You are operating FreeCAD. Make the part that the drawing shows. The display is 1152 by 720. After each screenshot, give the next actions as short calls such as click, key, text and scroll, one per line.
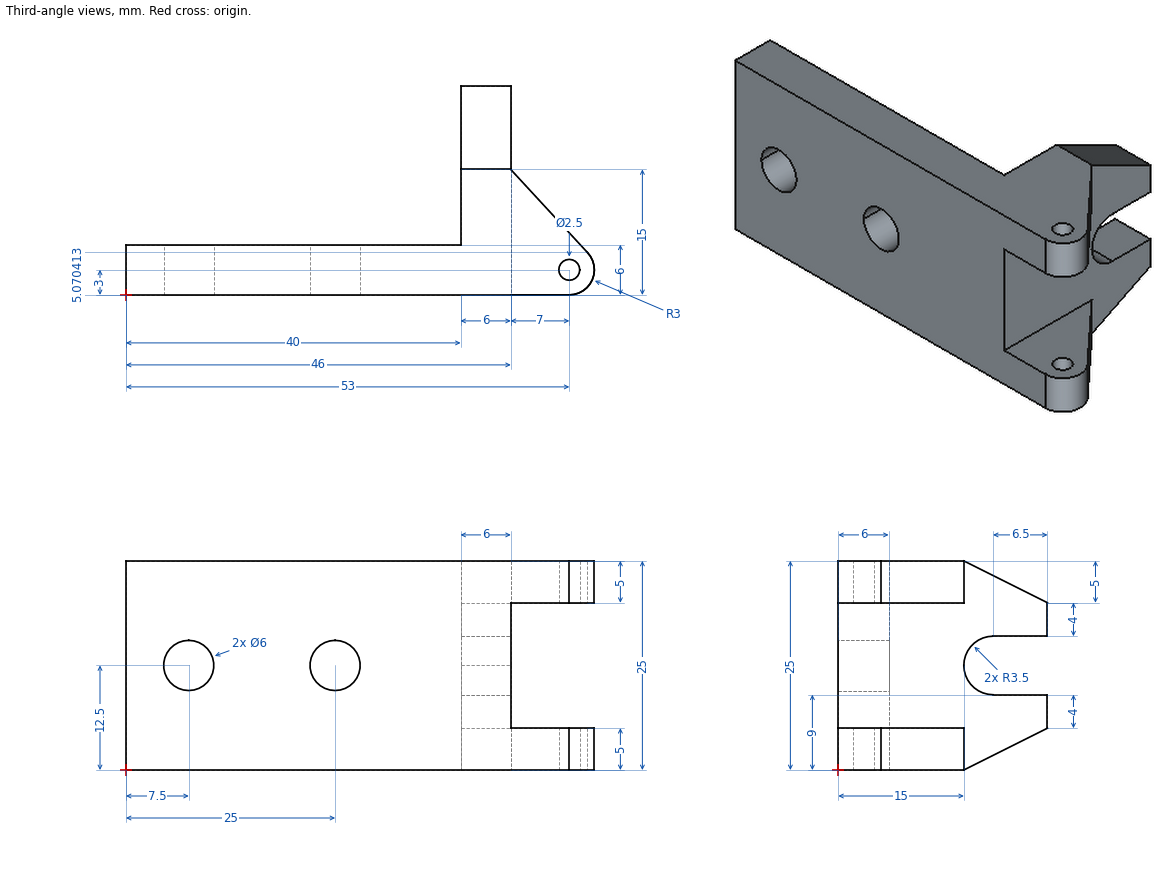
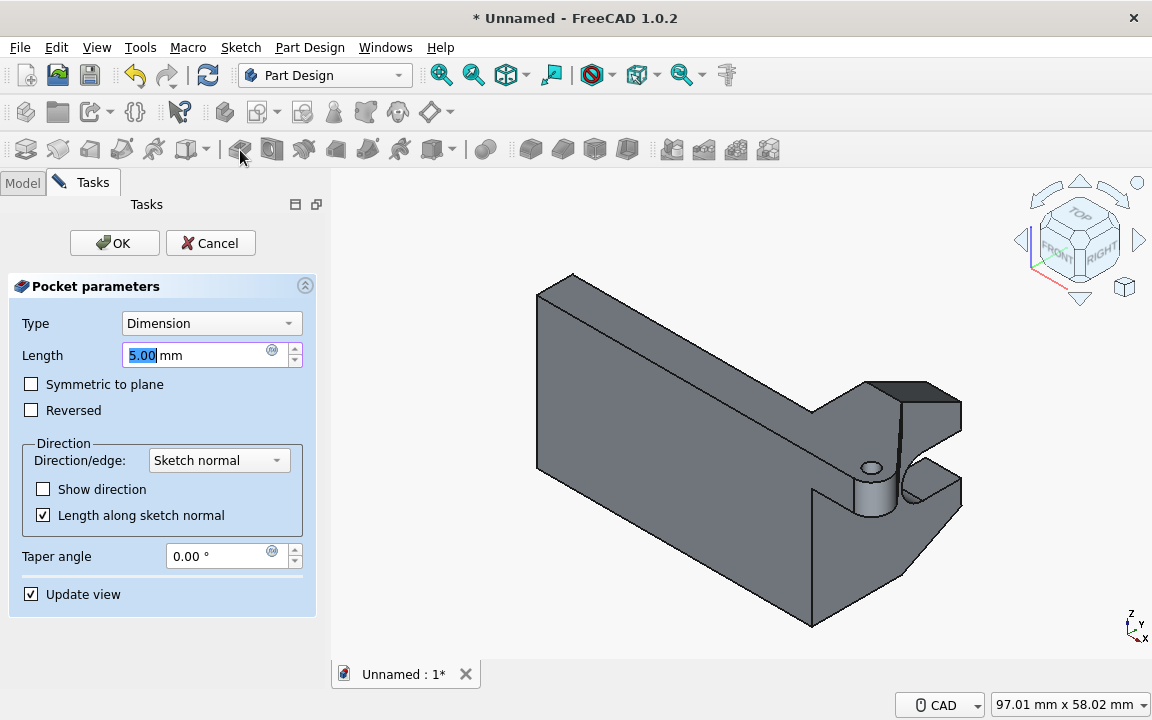
text(5)
key(Tab)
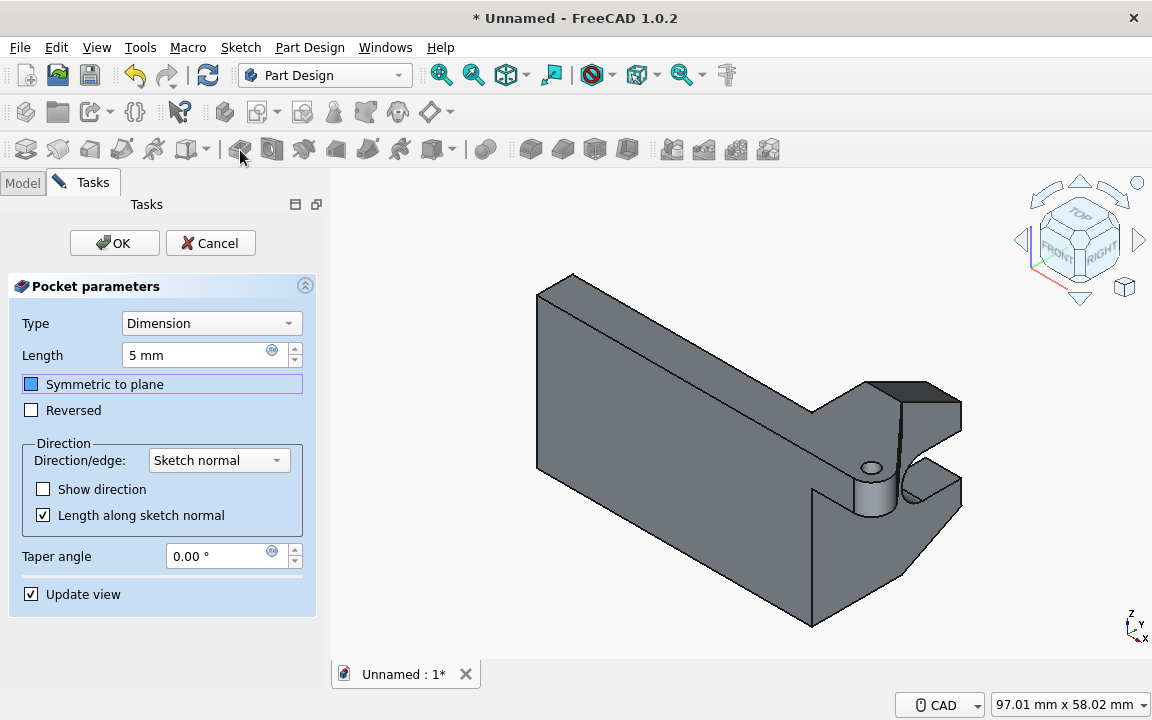
click(115, 243)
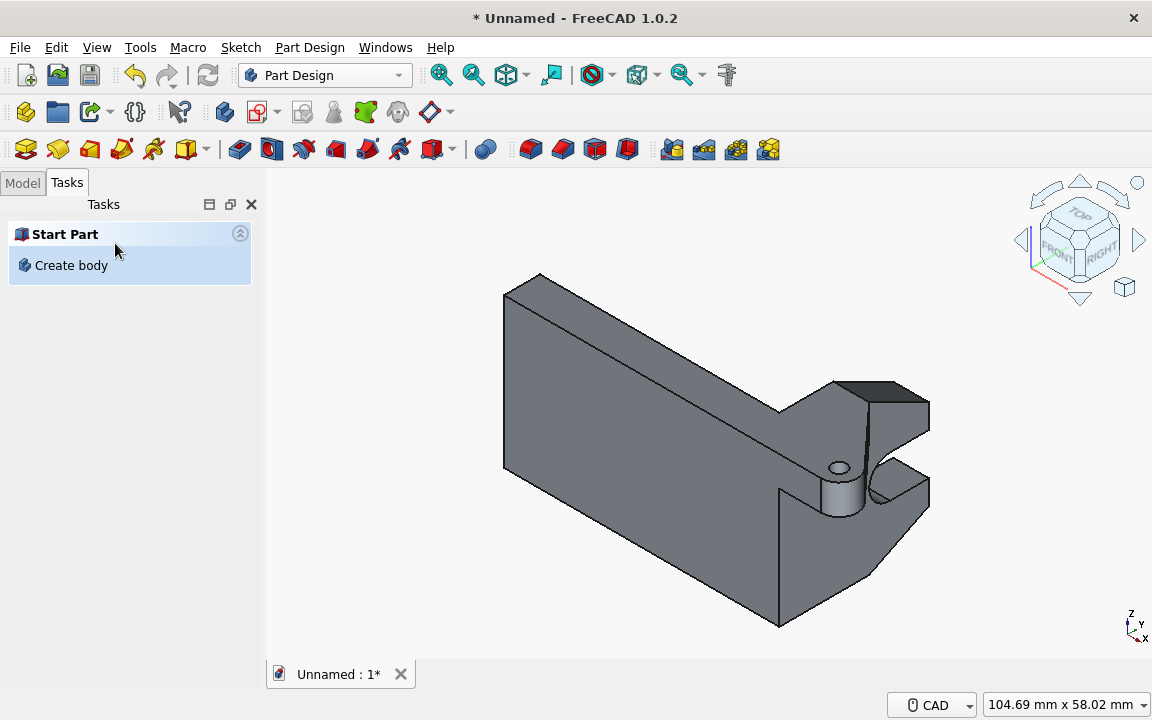
key(v)
key(f)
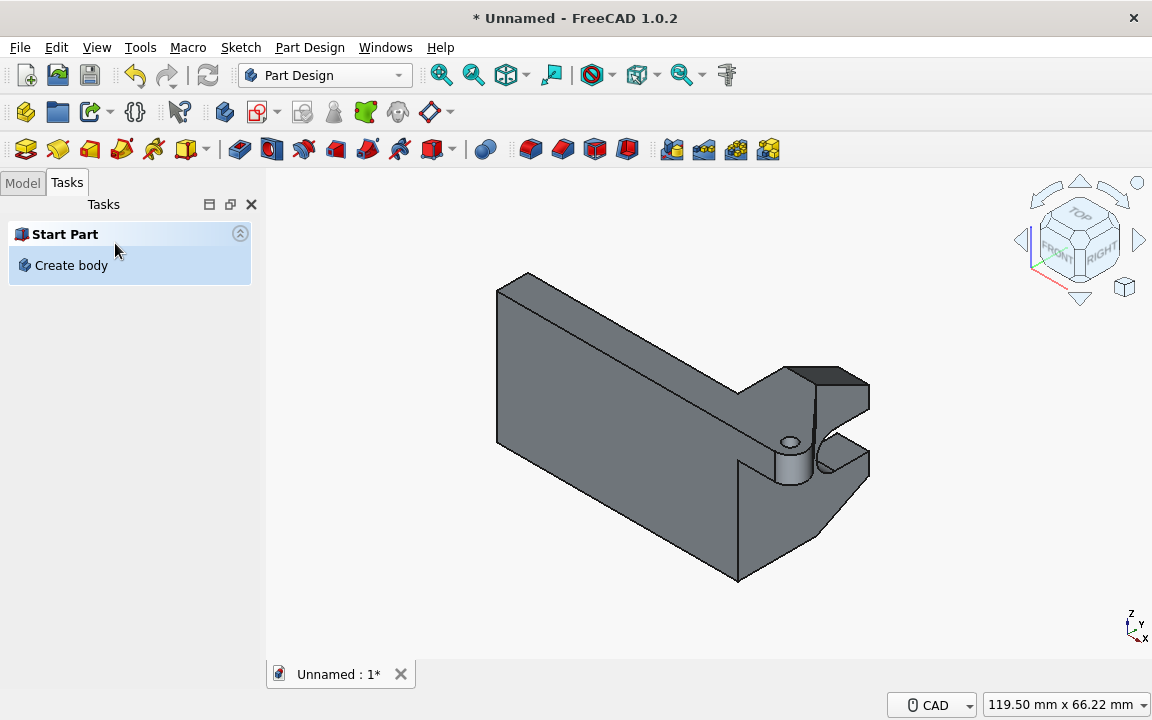
click(23, 182)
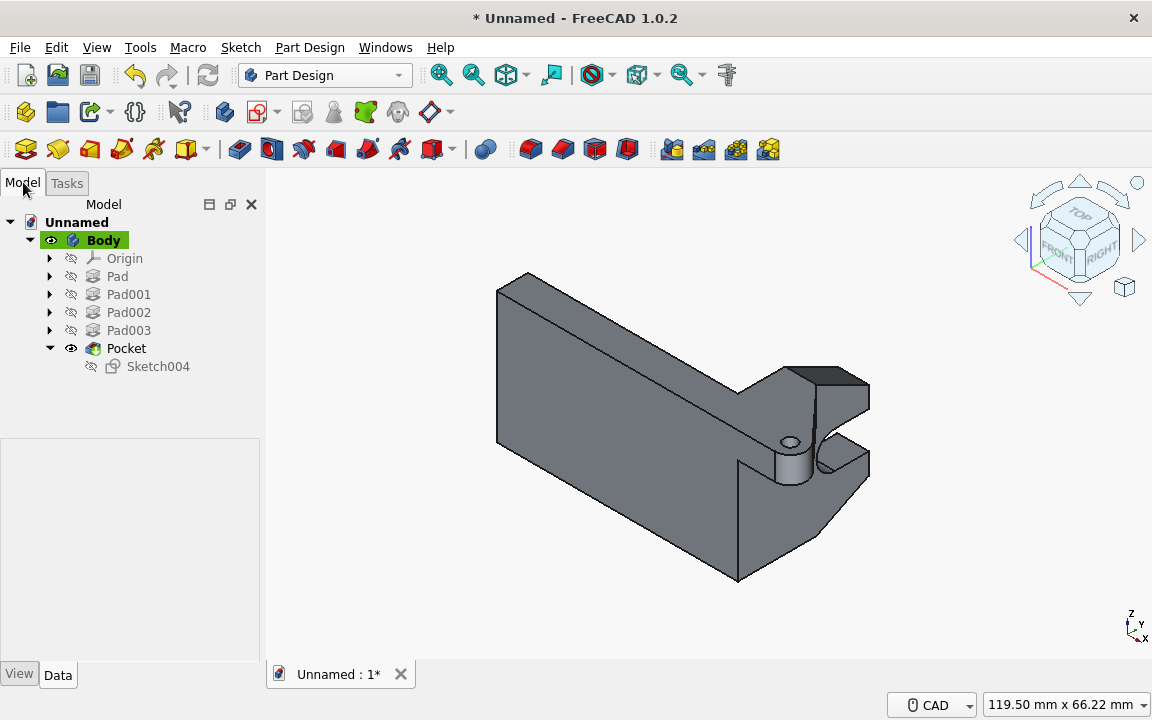
click(50, 258)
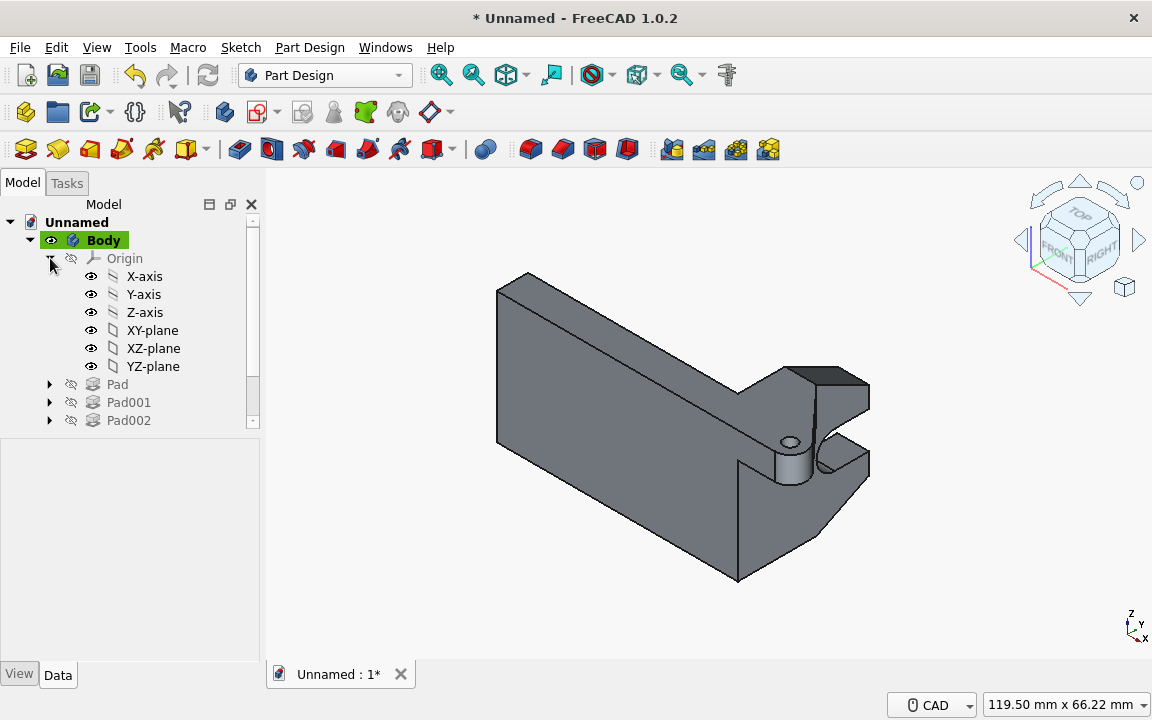
click(136, 330)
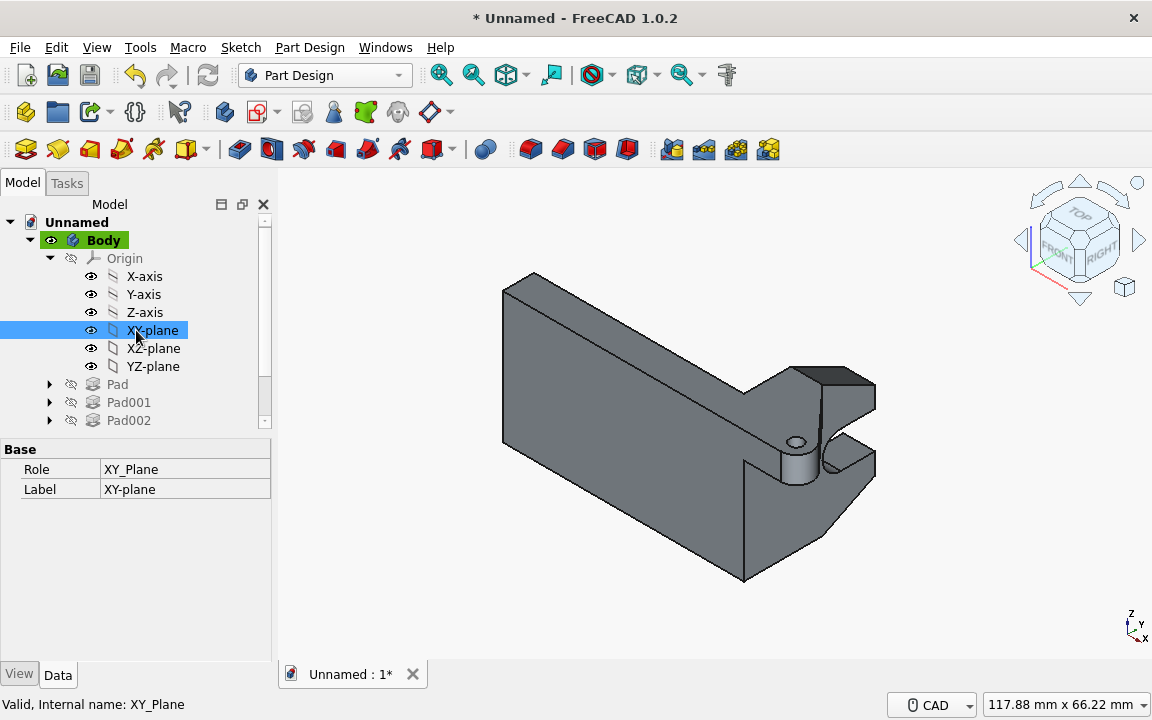
click(430, 112)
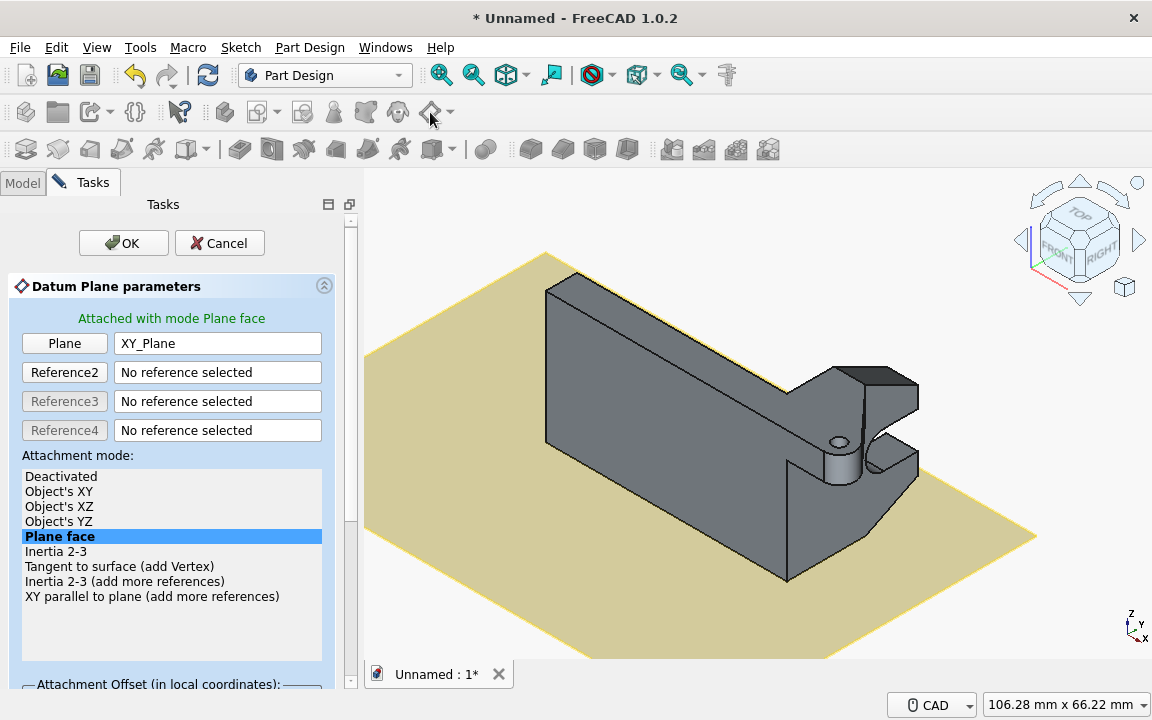
scroll(351, 451, down, 3)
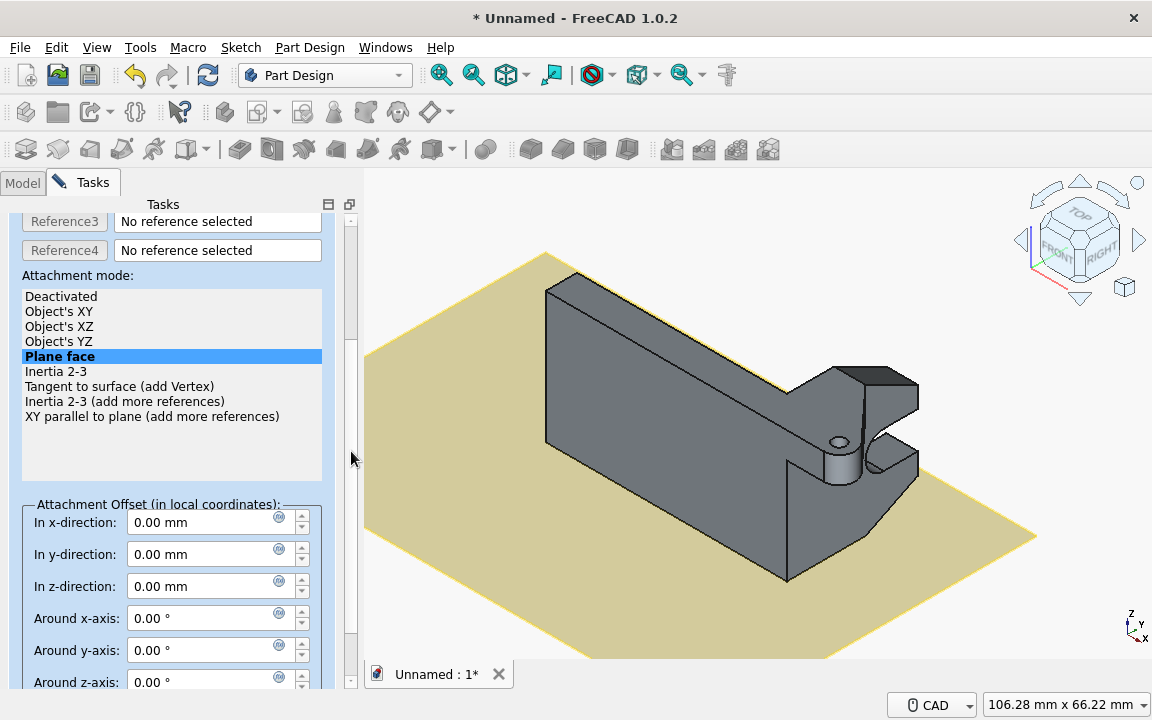
triple_click(210, 586)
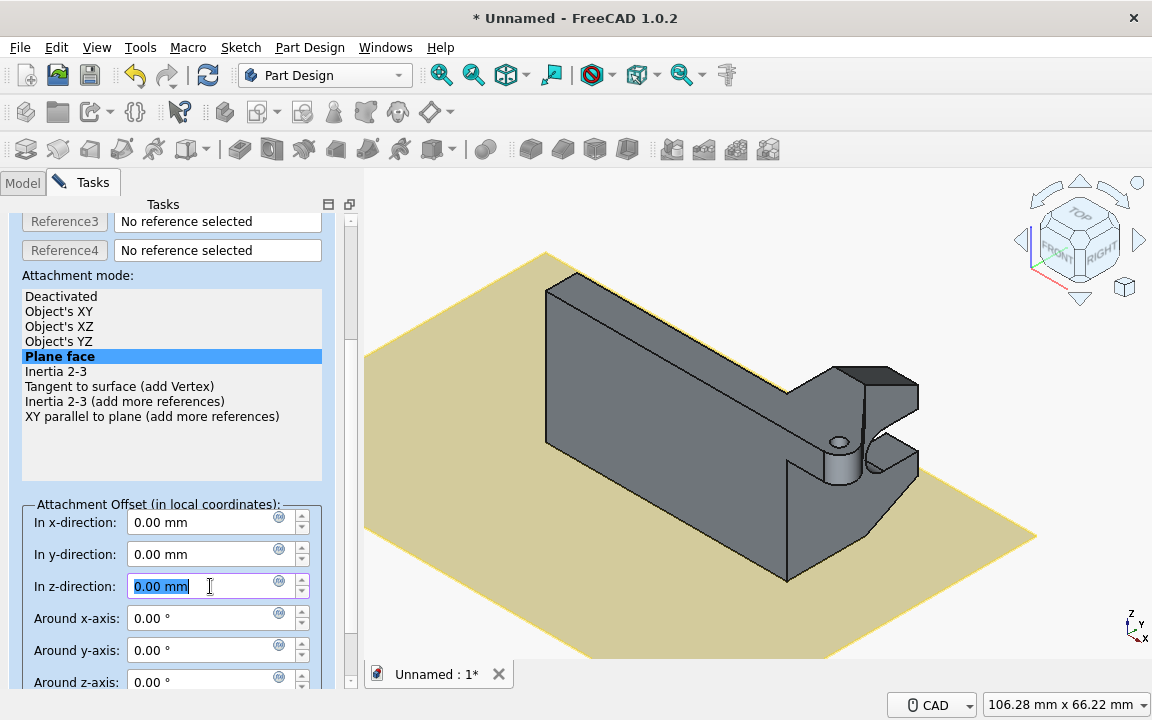
text(5)
key(Tab)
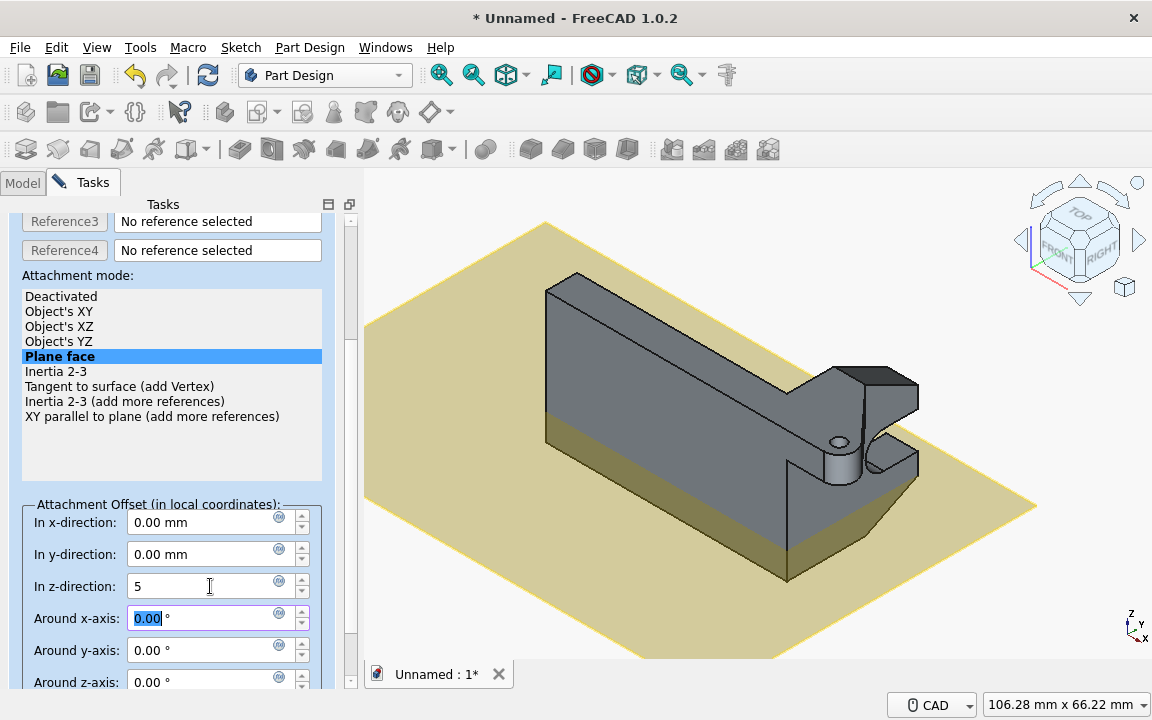
scroll(351, 451, up, 4)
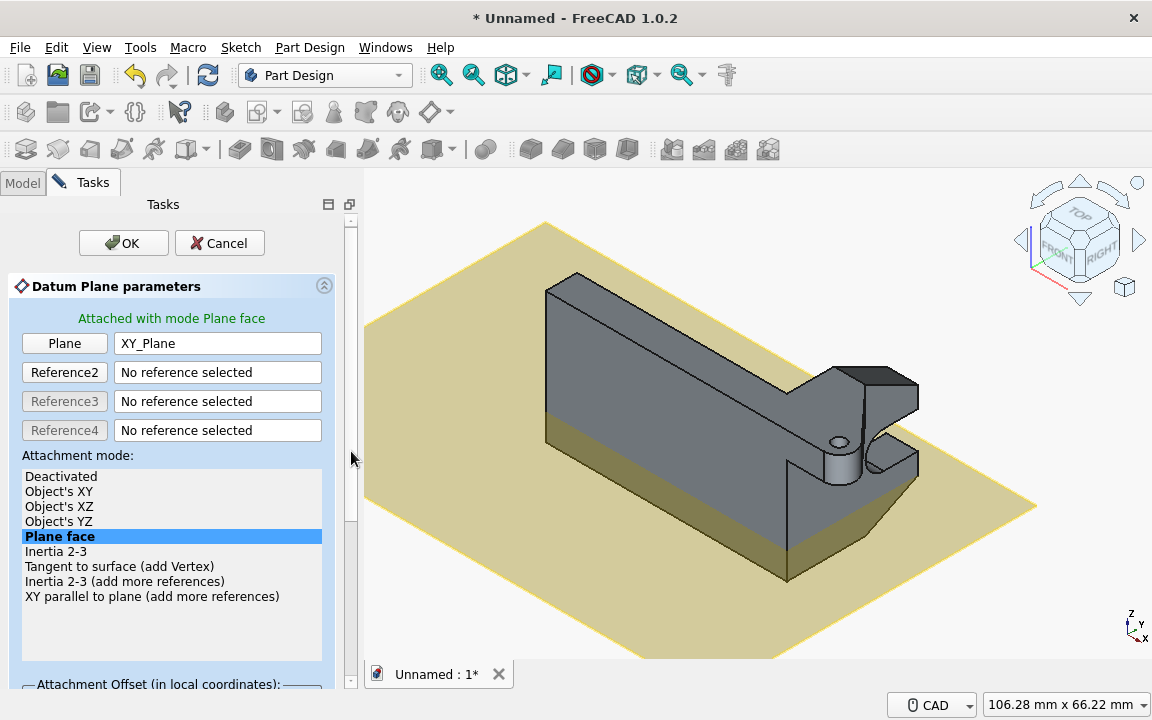
click(124, 243)